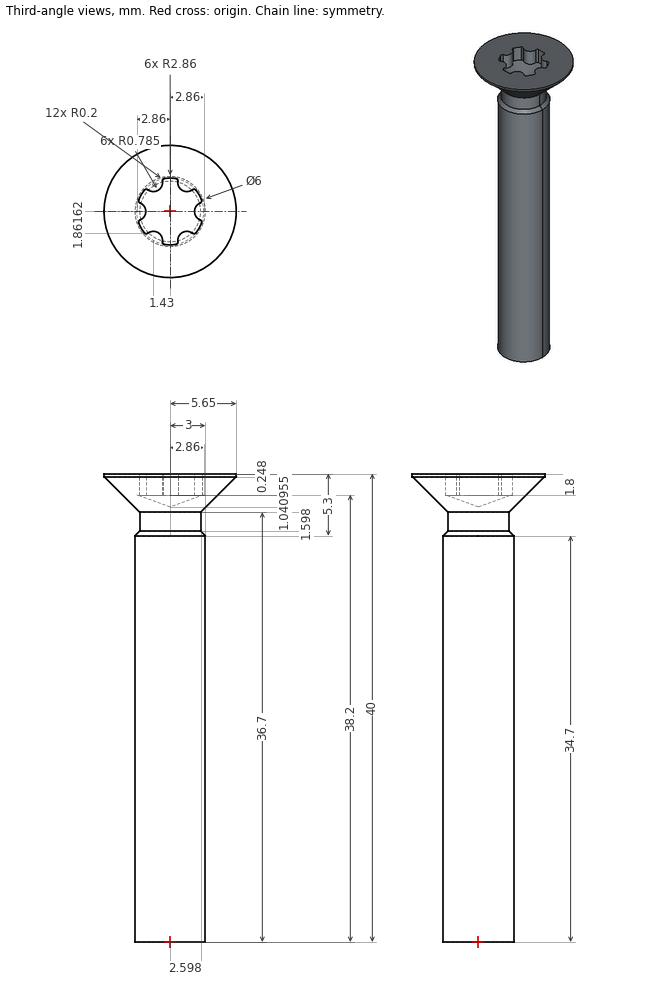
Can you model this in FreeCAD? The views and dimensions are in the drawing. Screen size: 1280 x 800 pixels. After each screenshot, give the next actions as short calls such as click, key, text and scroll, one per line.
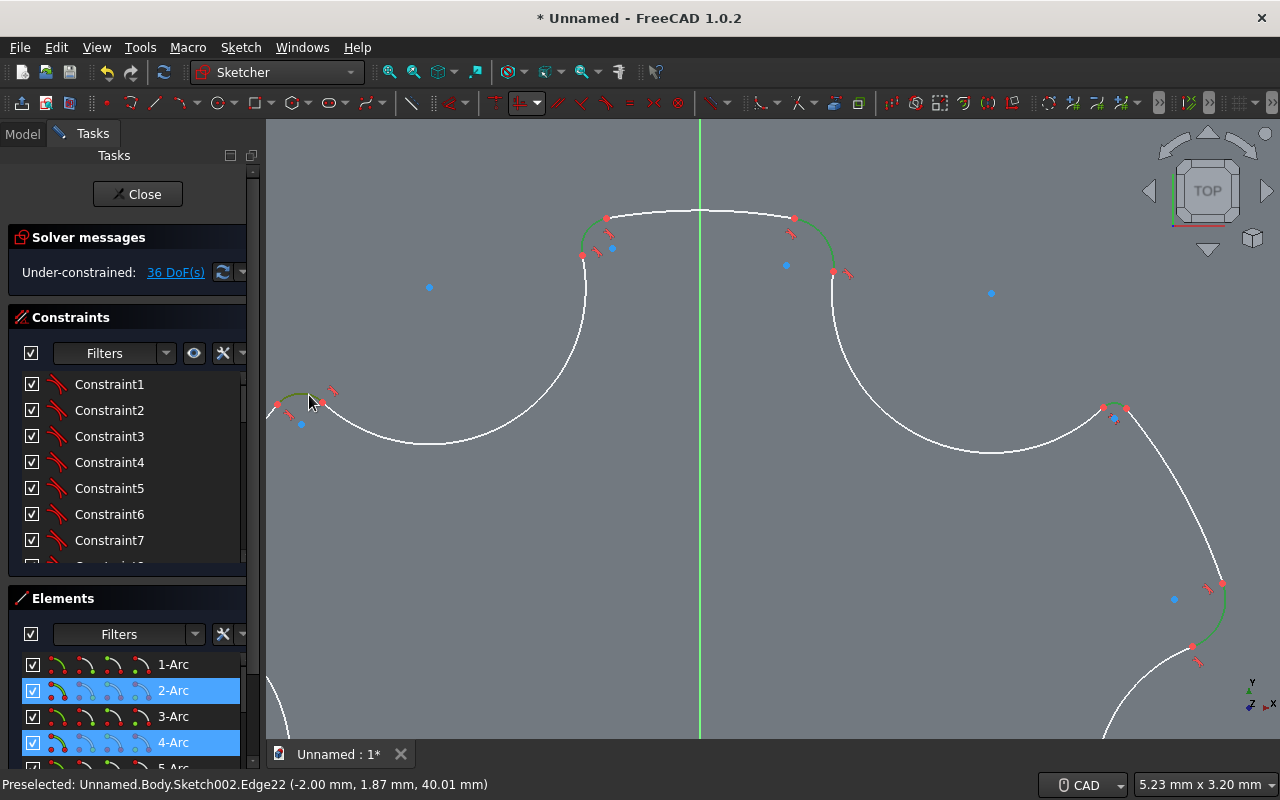
scroll(707, 237, down, 5)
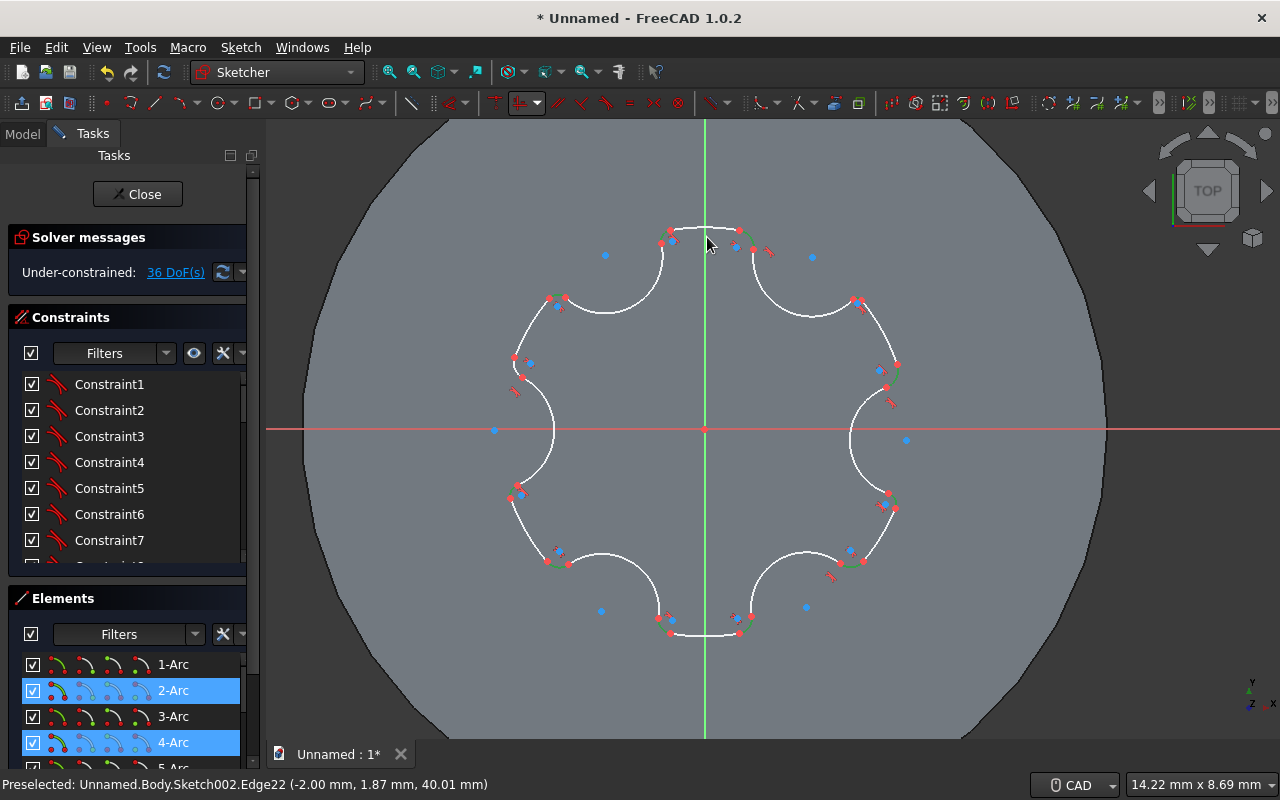
scroll(514, 364, up, 4)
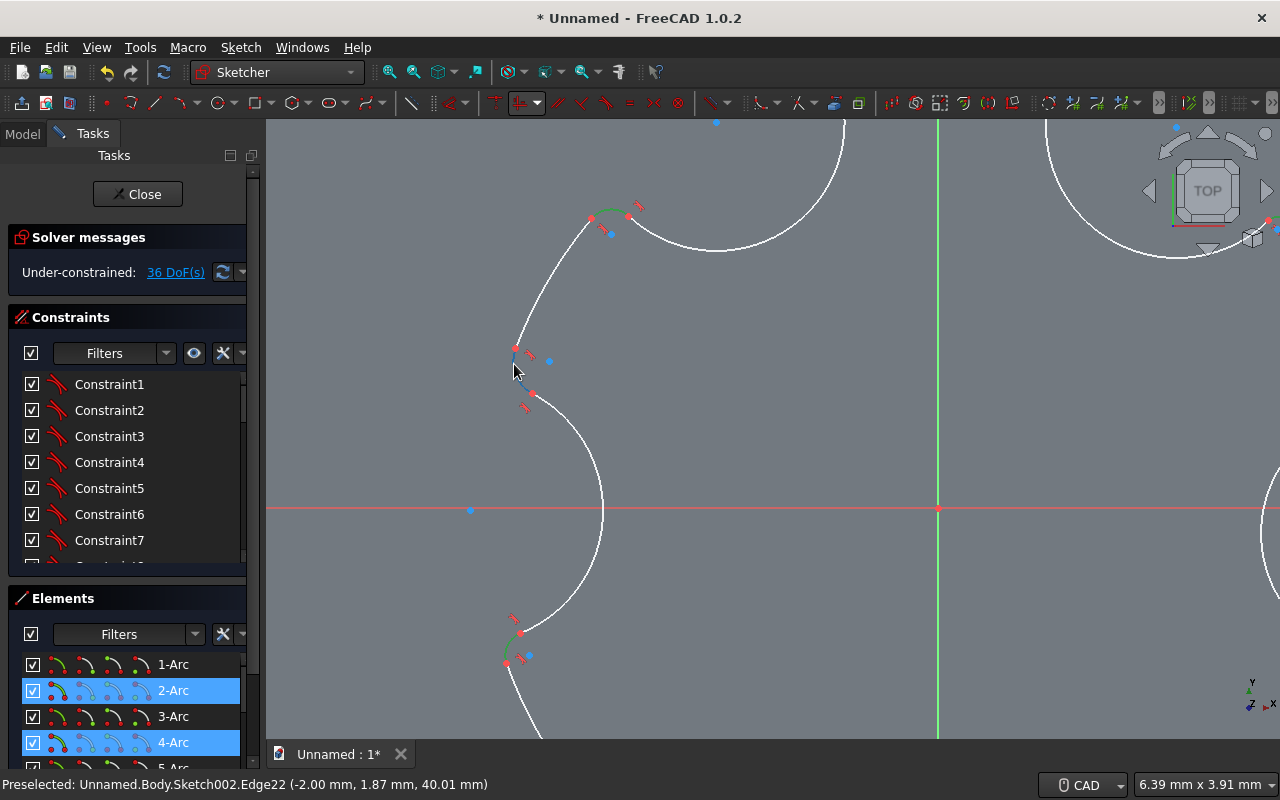
click(514, 364)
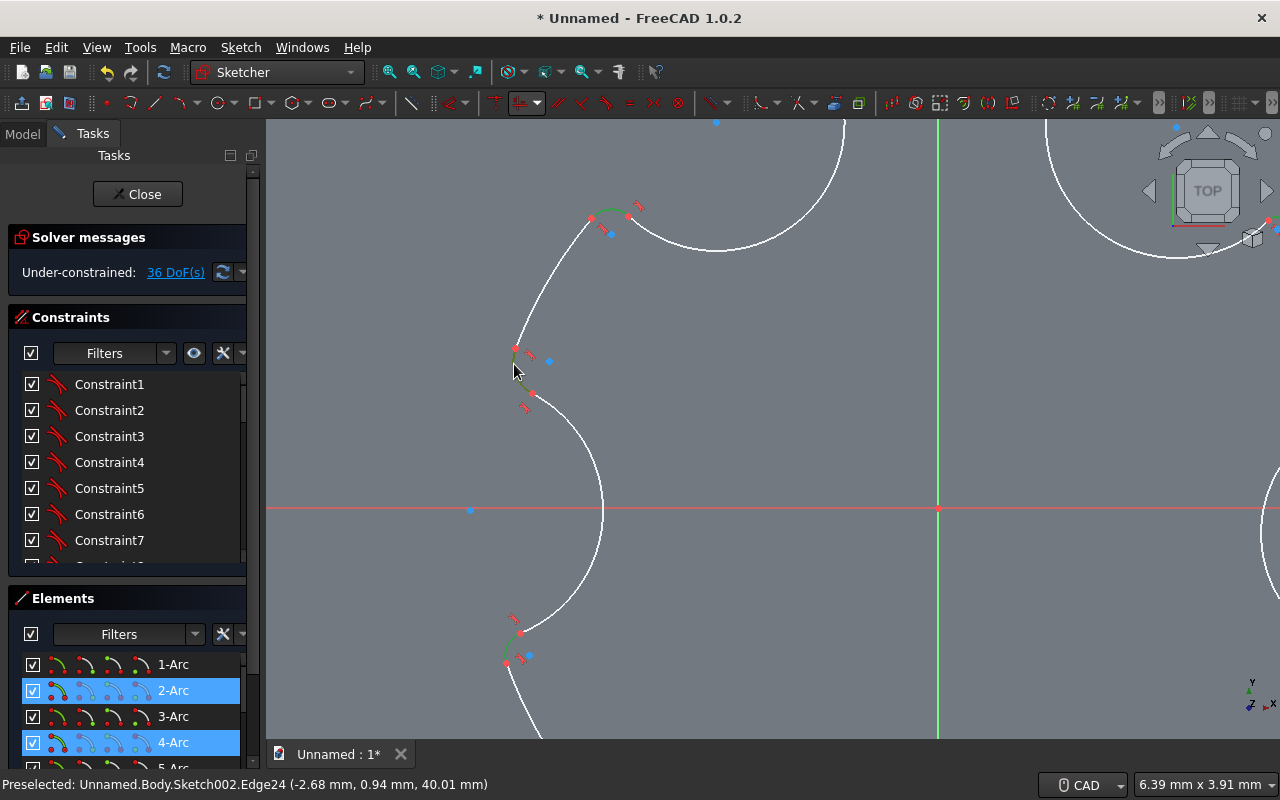
click(630, 104)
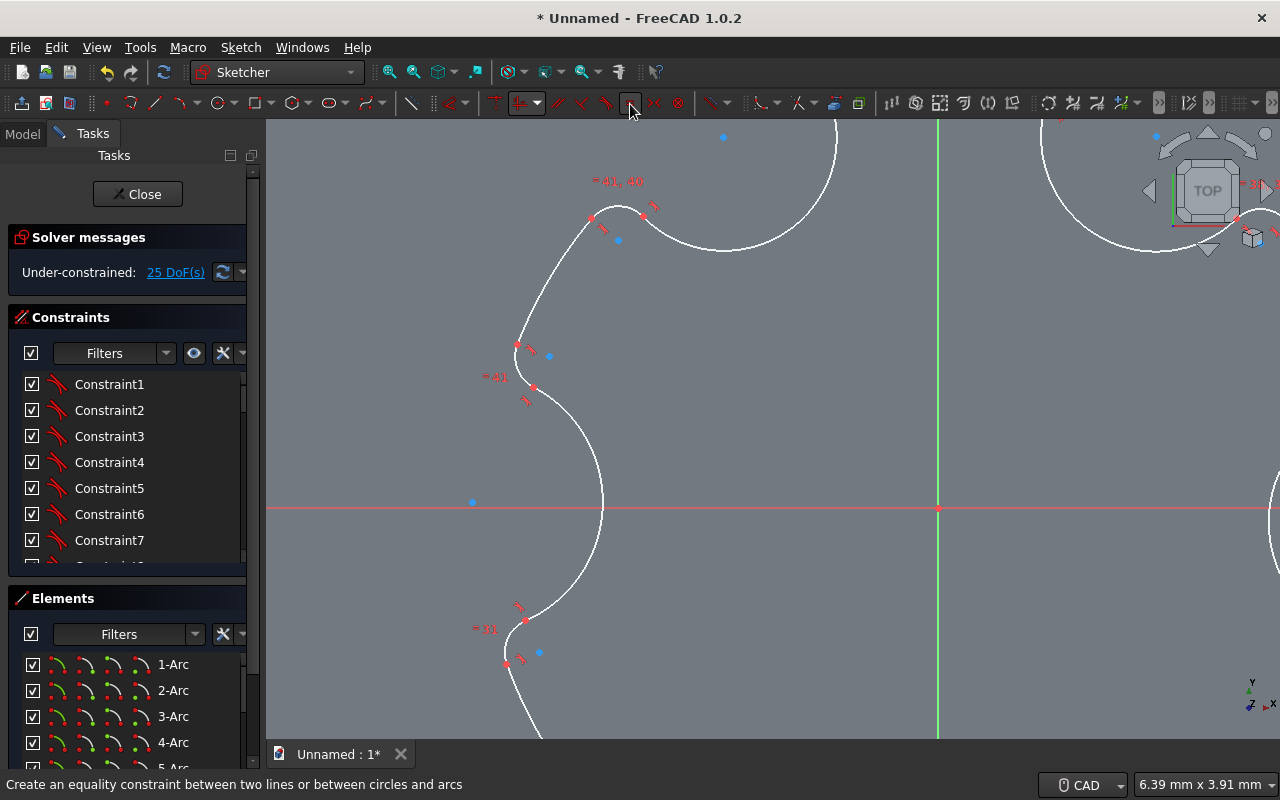
click(588, 562)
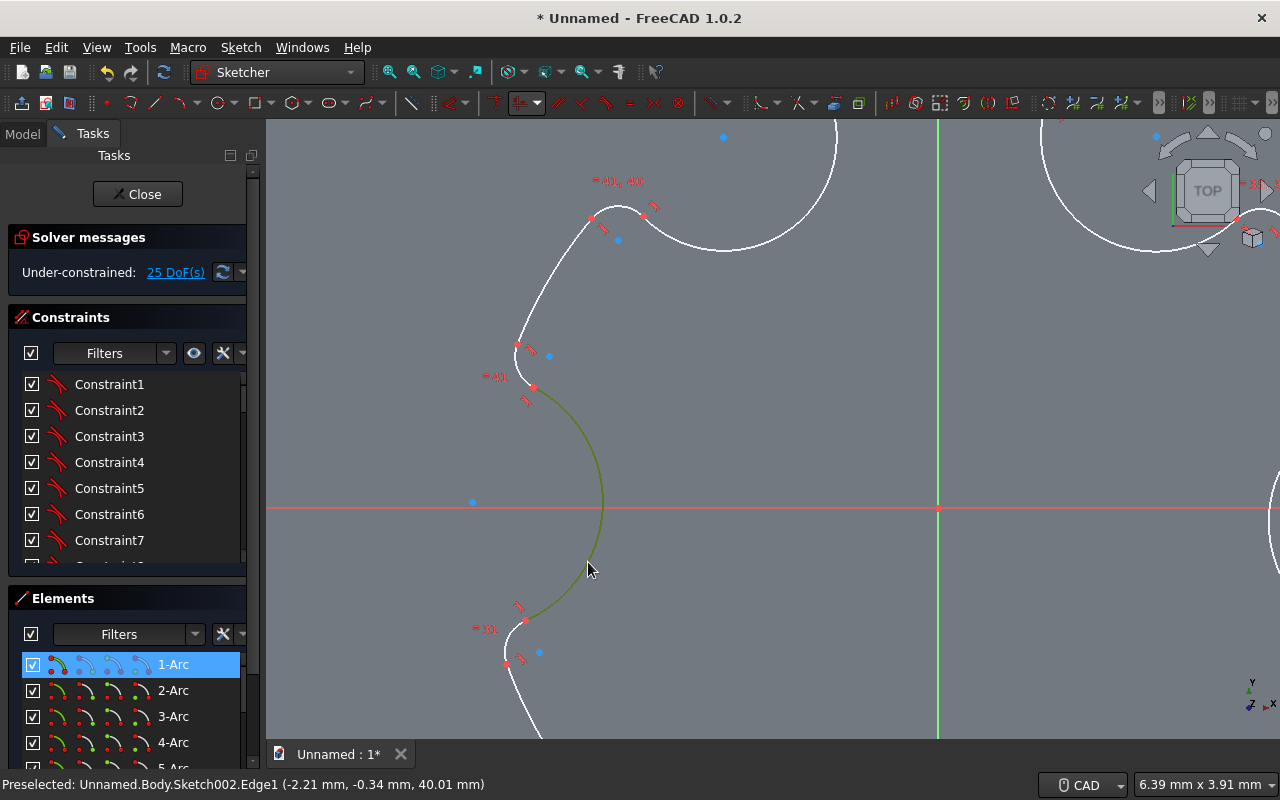
scroll(514, 364, down, 4)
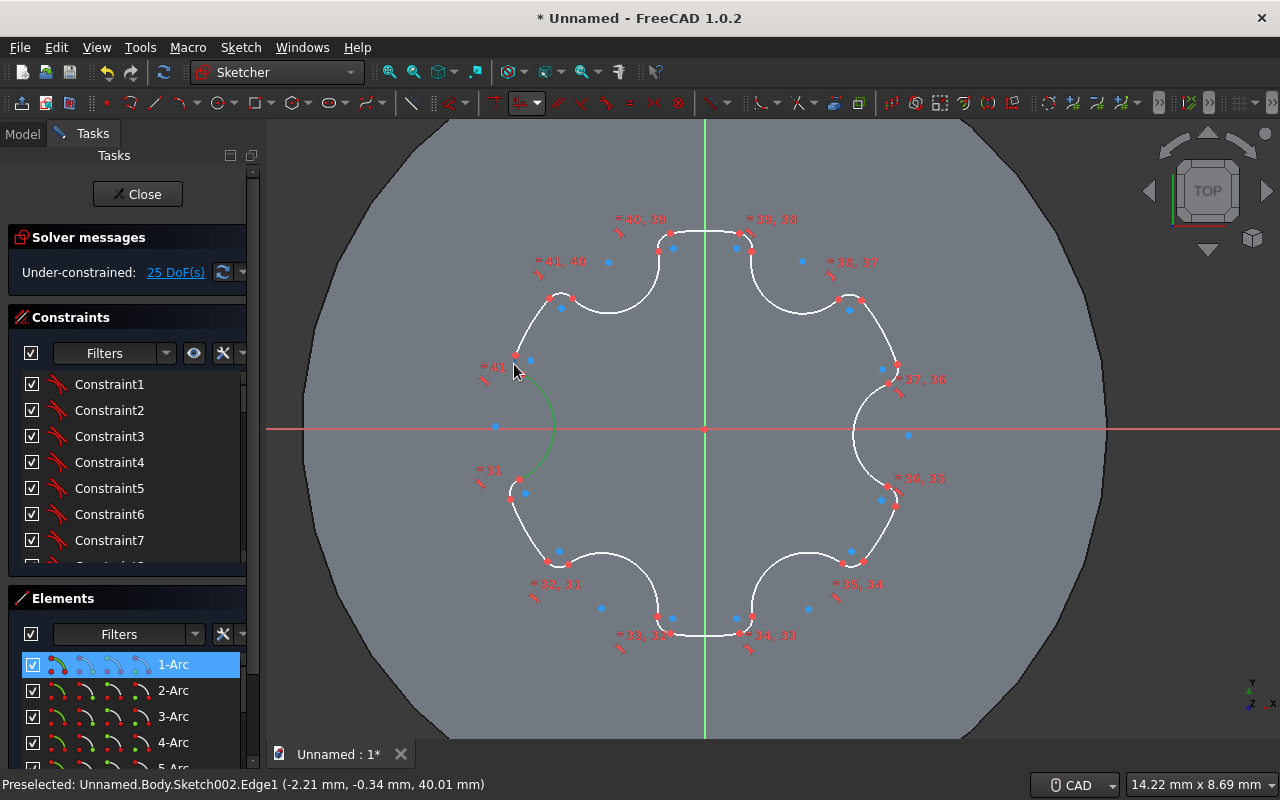
click(649, 579)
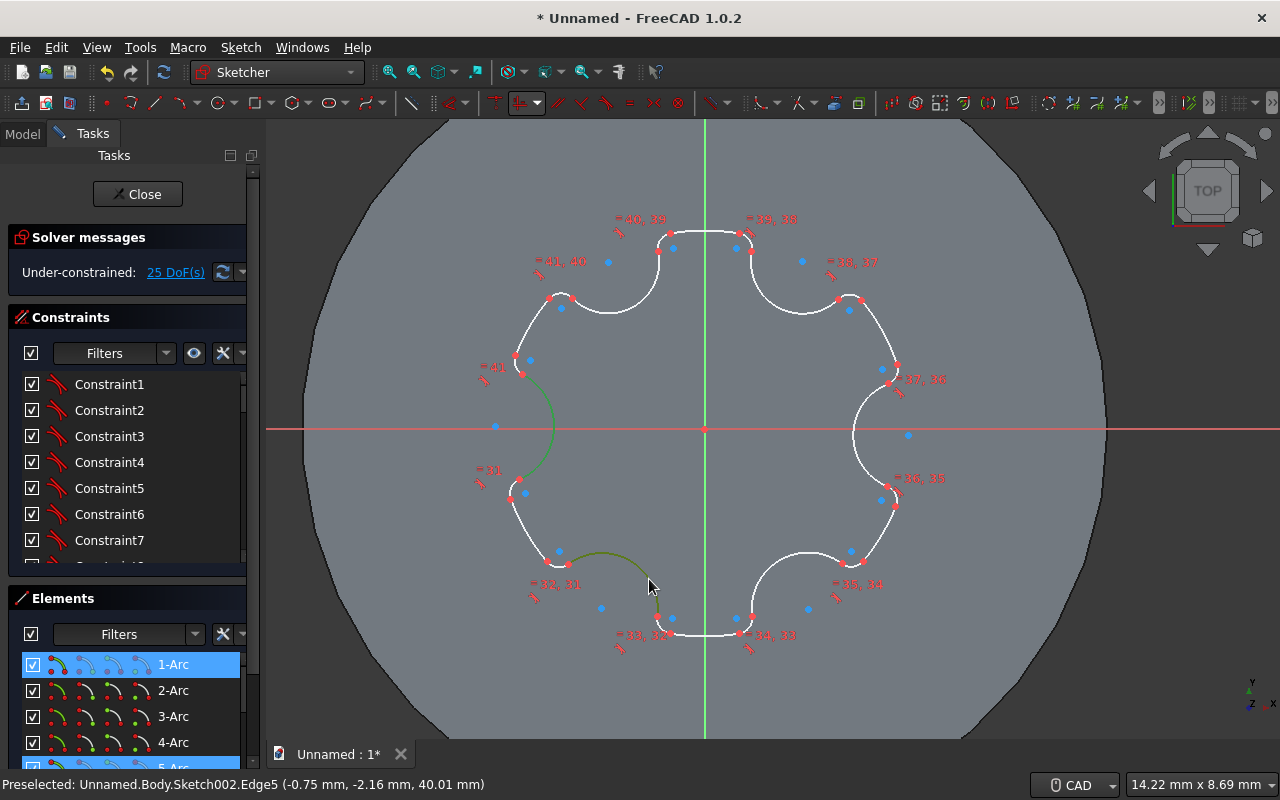
click(805, 553)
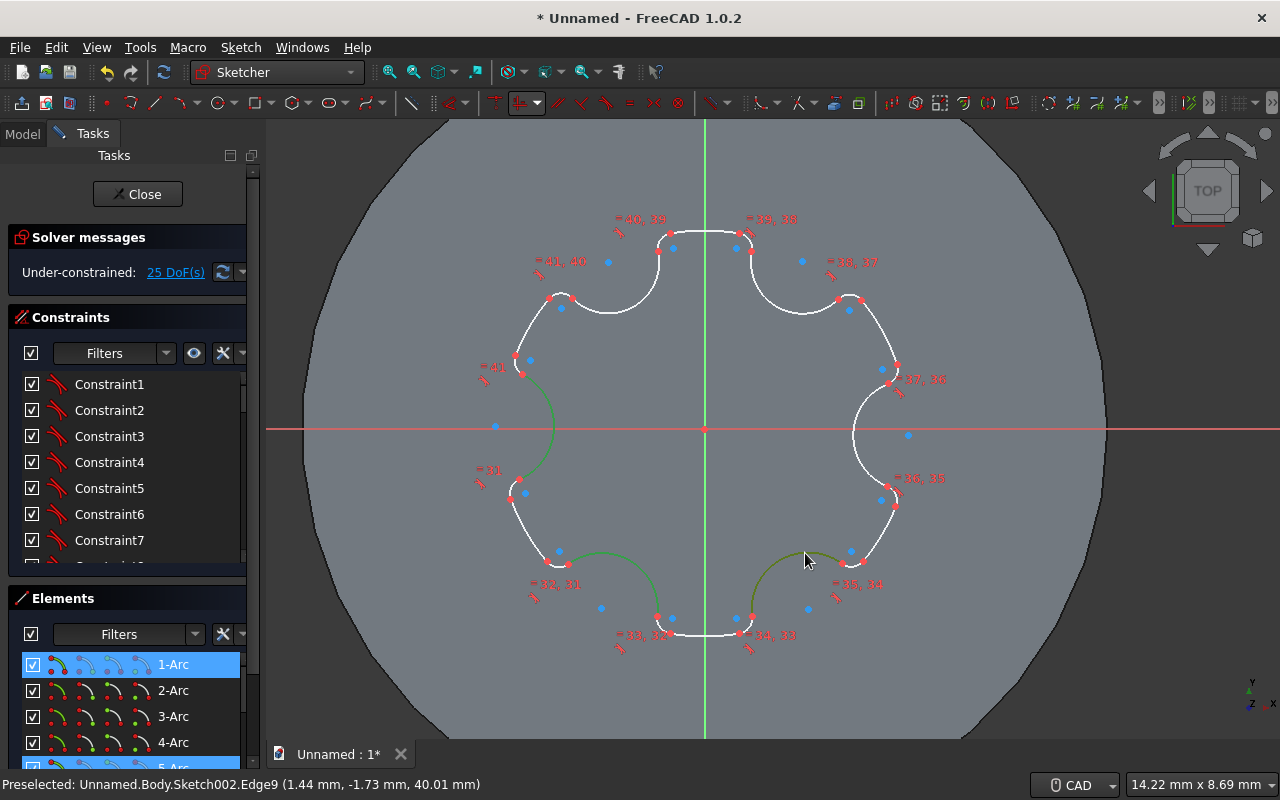
click(860, 410)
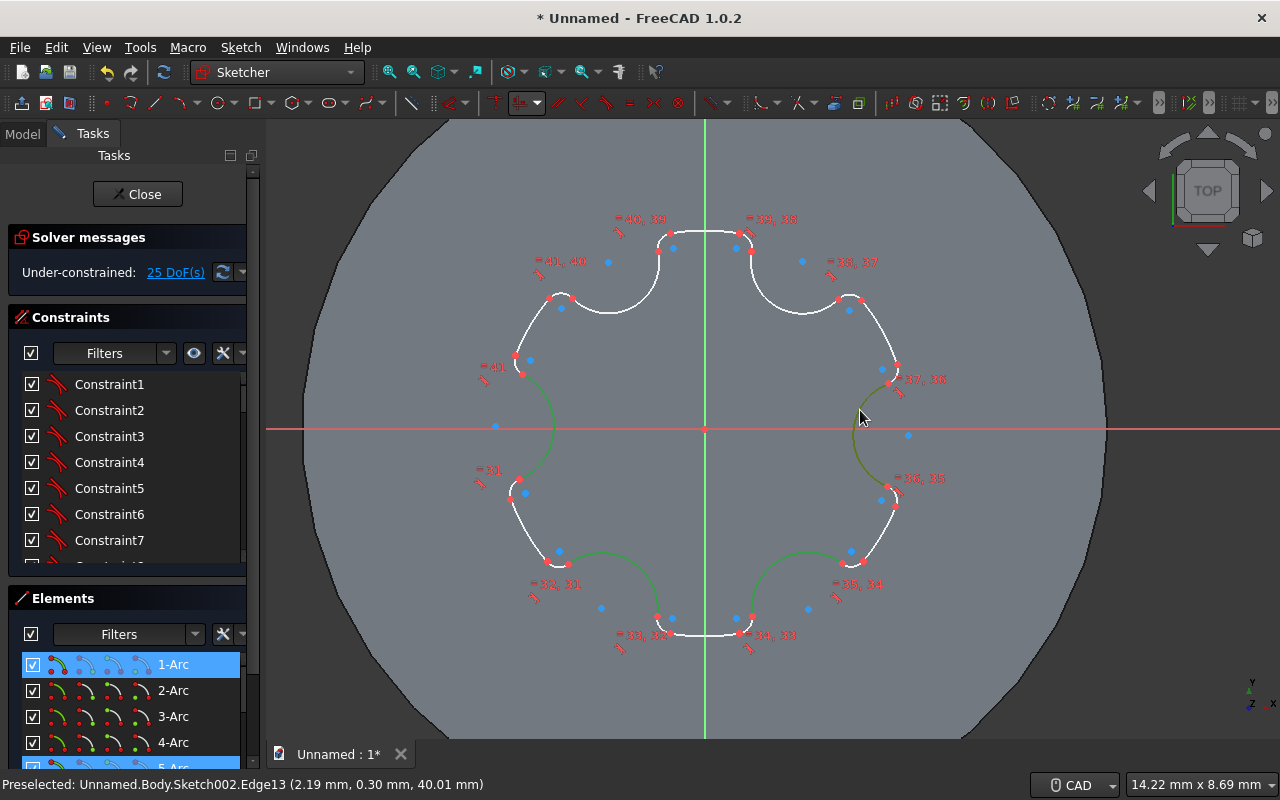
click(759, 290)